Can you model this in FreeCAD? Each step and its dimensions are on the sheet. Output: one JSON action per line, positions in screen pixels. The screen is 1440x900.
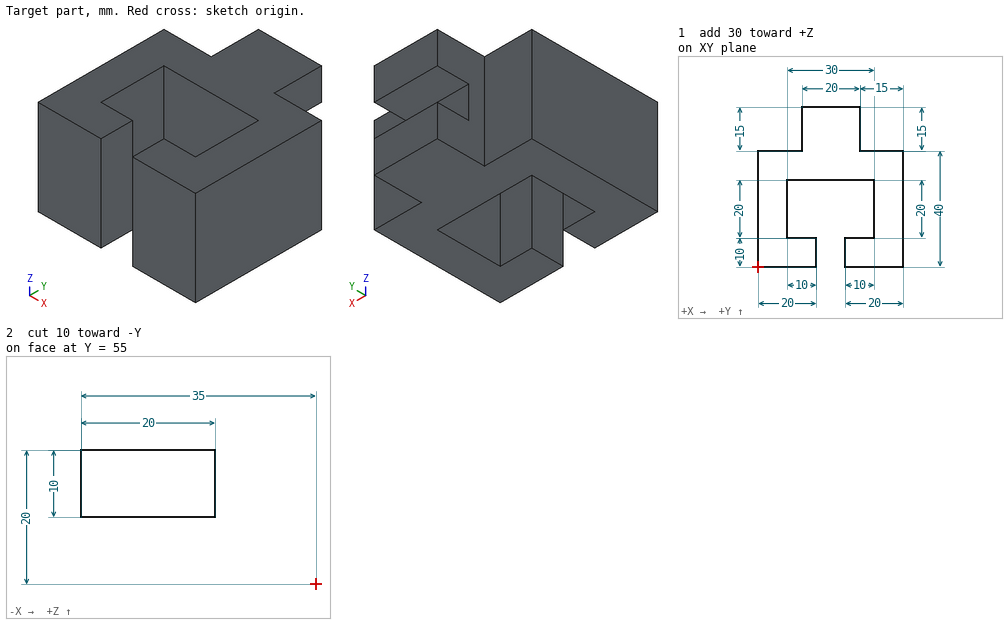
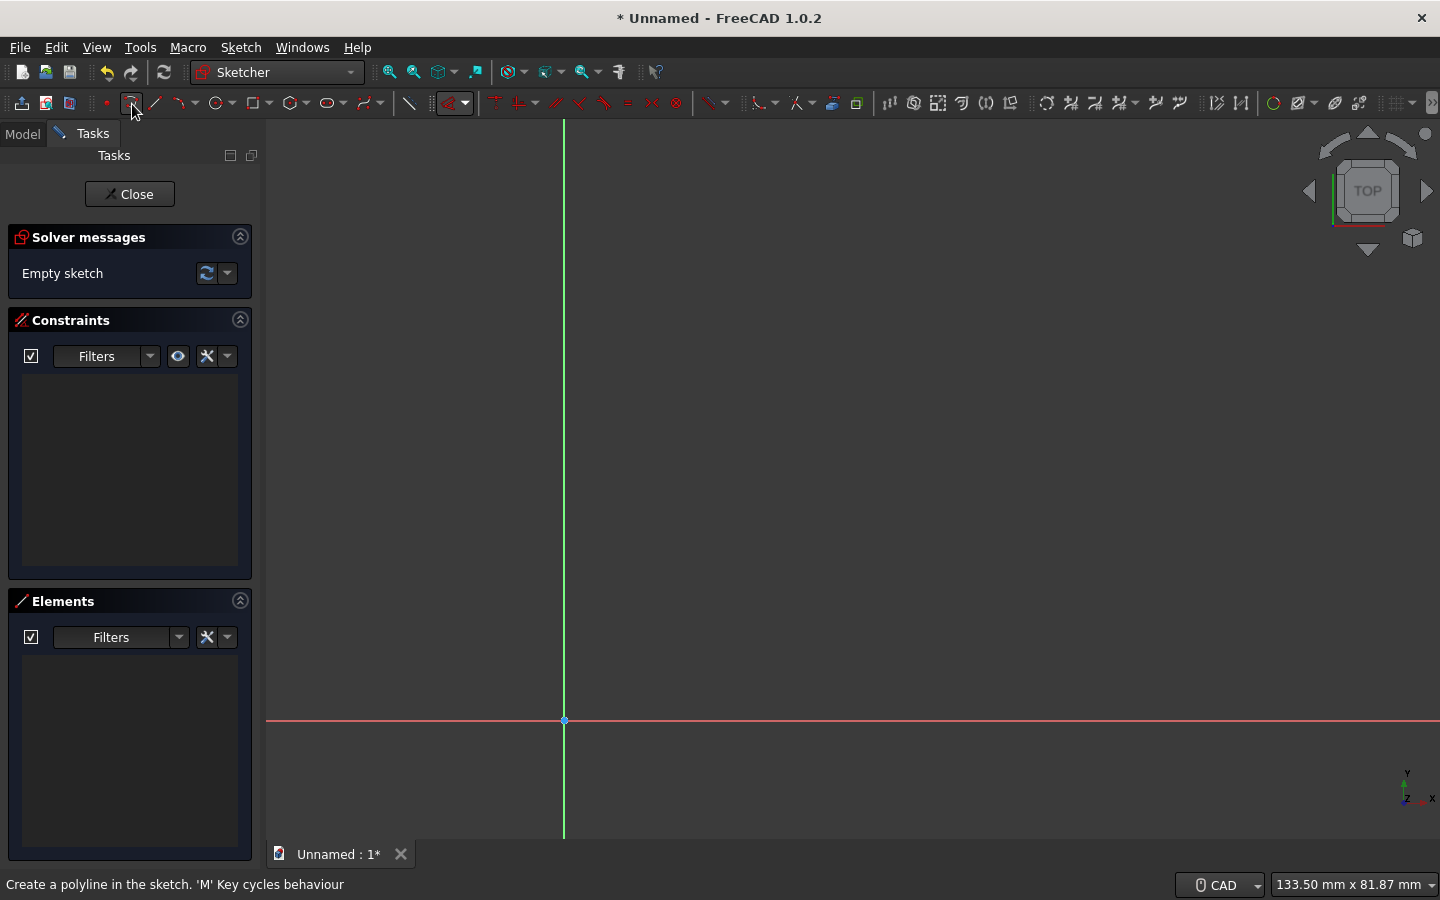
{"action": "left_click", "coordinate": [564, 721]}
{"action": "left_click", "coordinate": [740, 712]}
{"action": "left_click", "coordinate": [740, 633]}
{"action": "left_click", "coordinate": [652, 633]}
{"action": "left_click", "coordinate": [652, 457]}
{"action": "left_click", "coordinate": [916, 457]}
{"action": "left_click", "coordinate": [916, 633]}
{"action": "left_click", "coordinate": [828, 633]}
{"action": "left_click", "coordinate": [828, 721]}
{"action": "left_click", "coordinate": [1004, 712]}
{"action": "left_click", "coordinate": [1004, 369]}
{"action": "left_click", "coordinate": [872, 369]}
{"action": "left_click", "coordinate": [872, 237]}
{"action": "left_click", "coordinate": [696, 237]}
{"action": "left_click", "coordinate": [696, 369]}
{"action": "left_click", "coordinate": [573, 369]}
{"action": "left_click", "coordinate": [564, 721]}
{"action": "key", "text": "Escape"}
{"action": "key", "text": "Escape"}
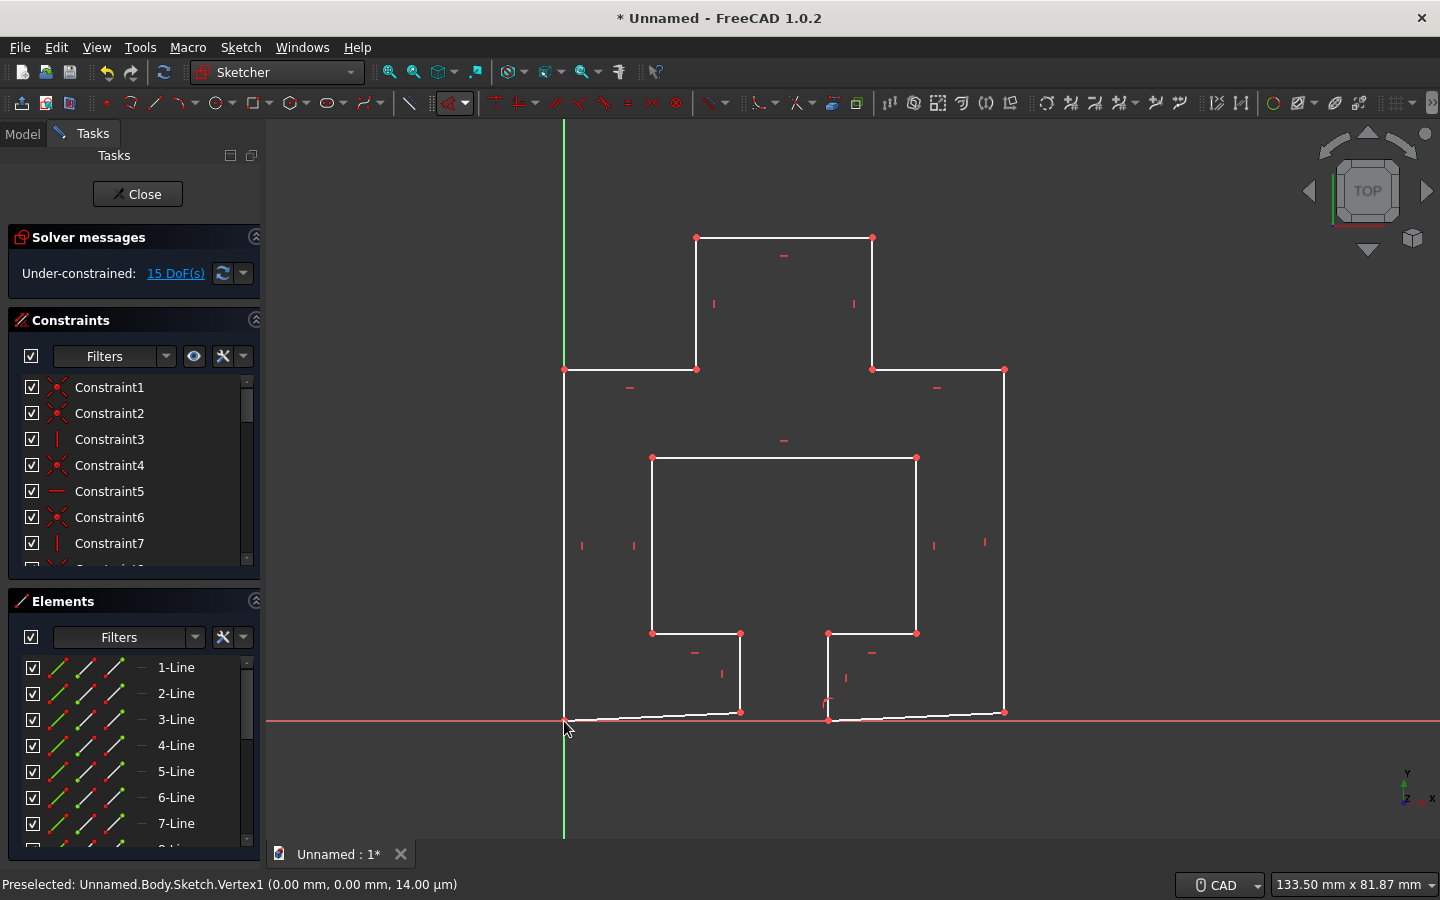
{"action": "left_click", "coordinate": [617, 719]}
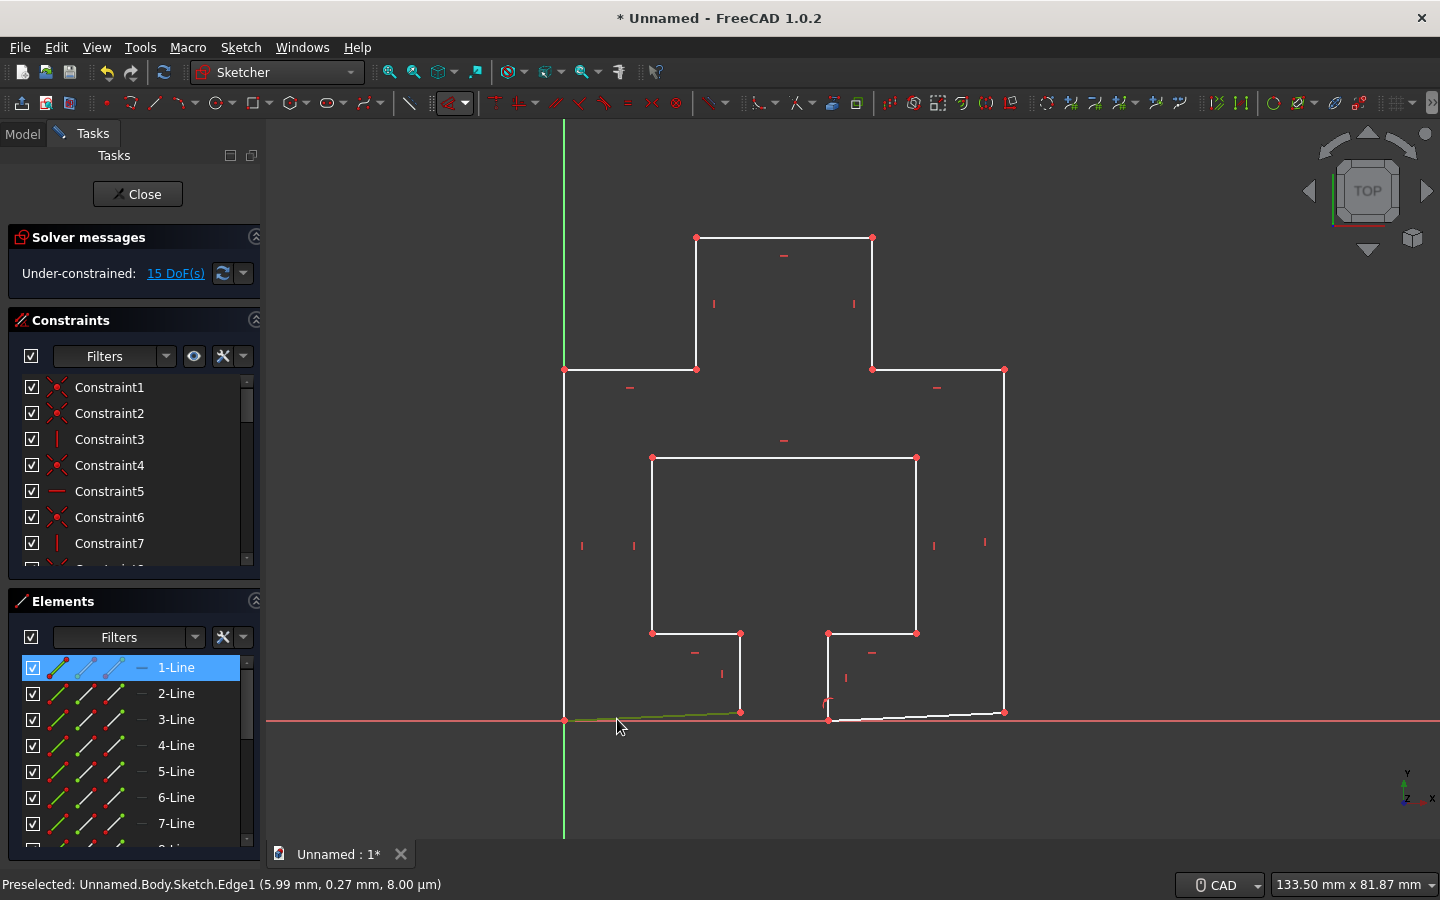
{"action": "key", "text": "h"}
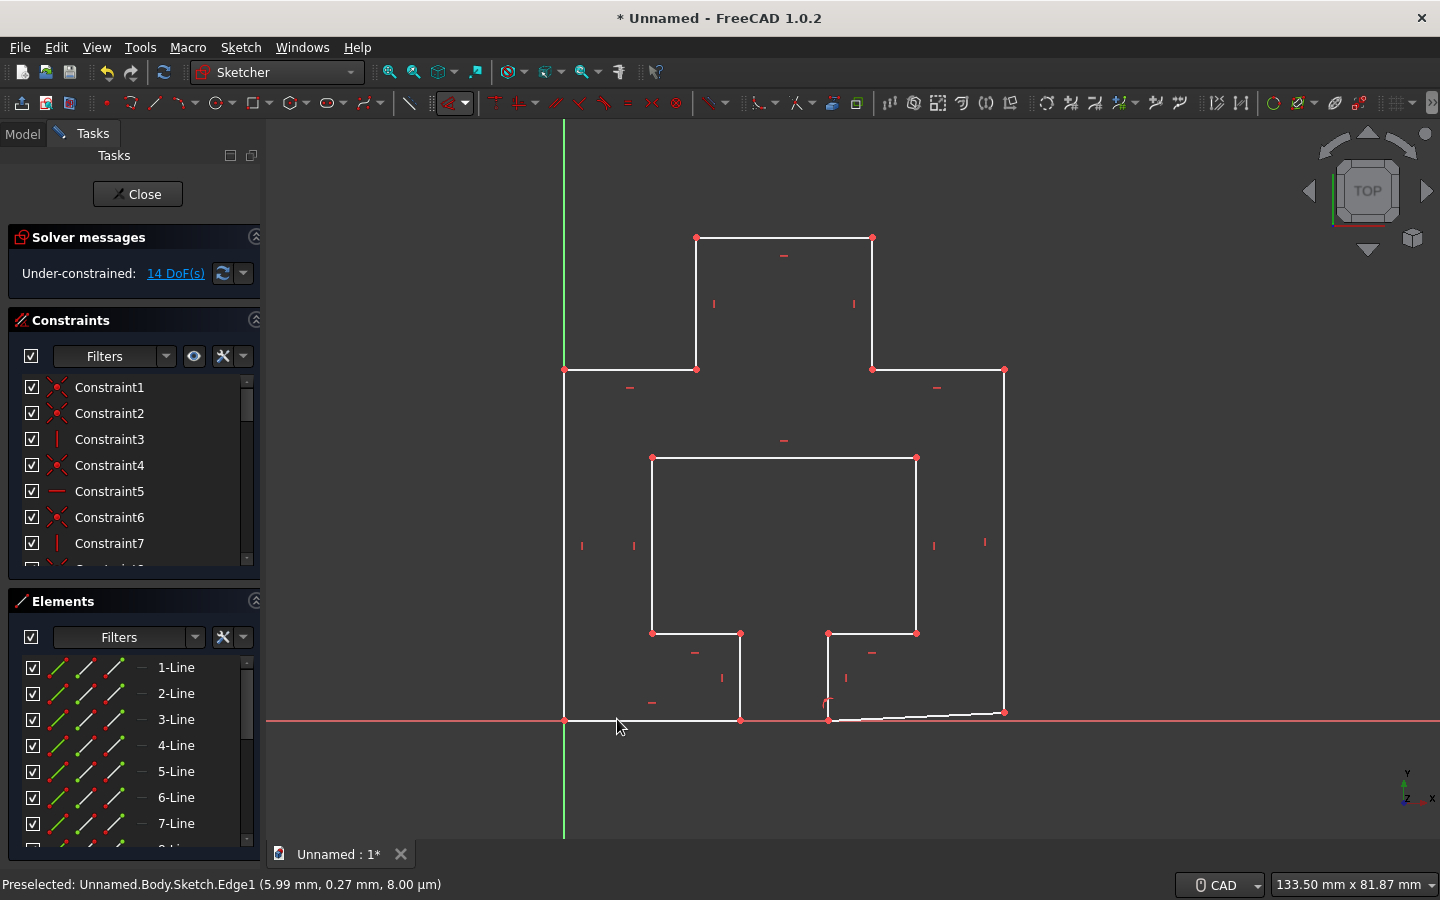
{"action": "left_click", "coordinate": [881, 719]}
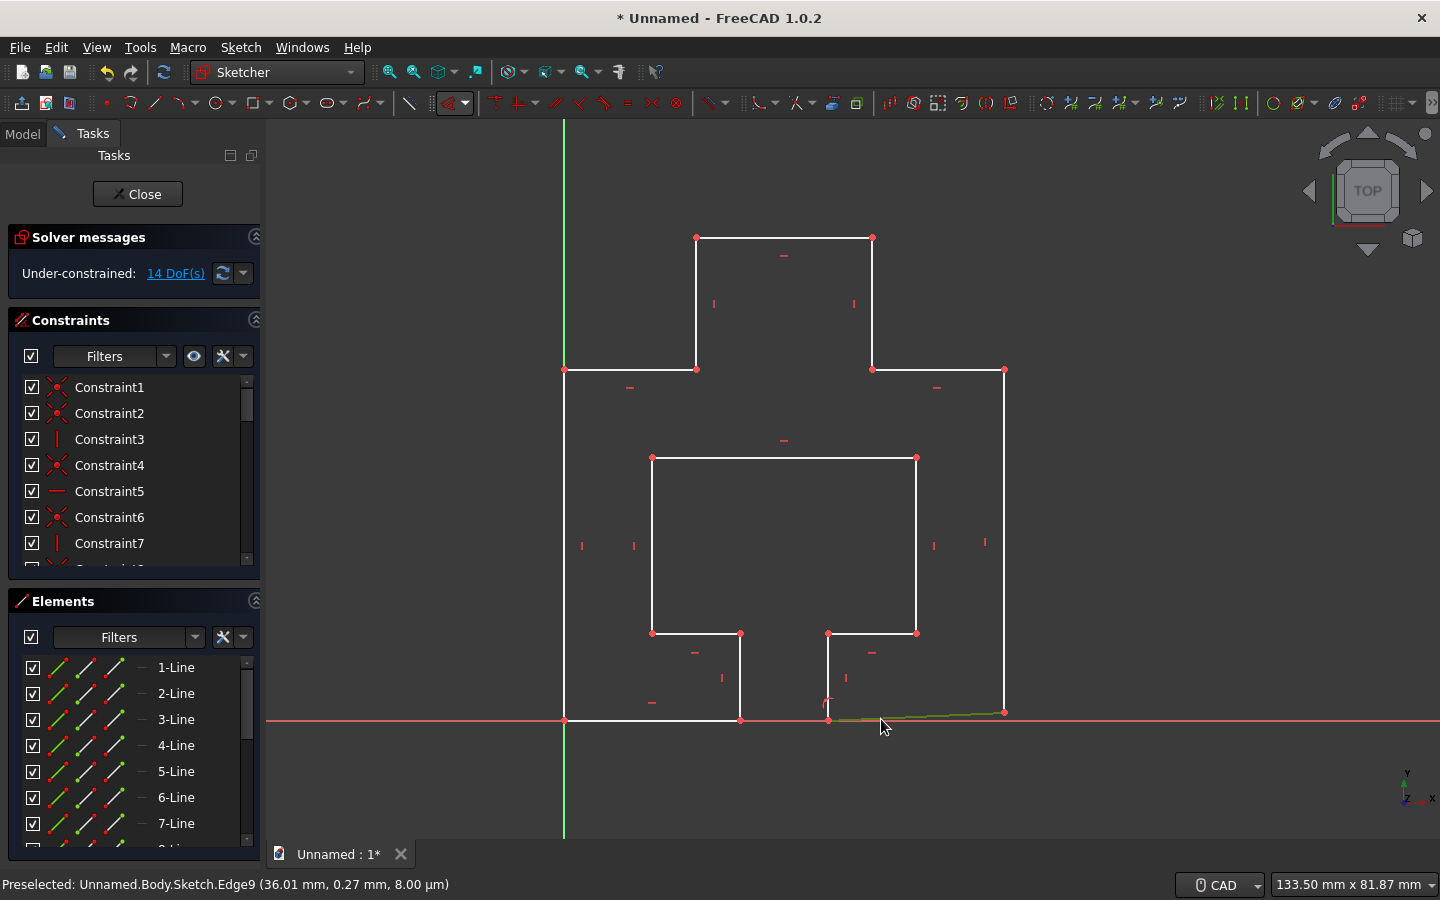
{"action": "key", "text": "h"}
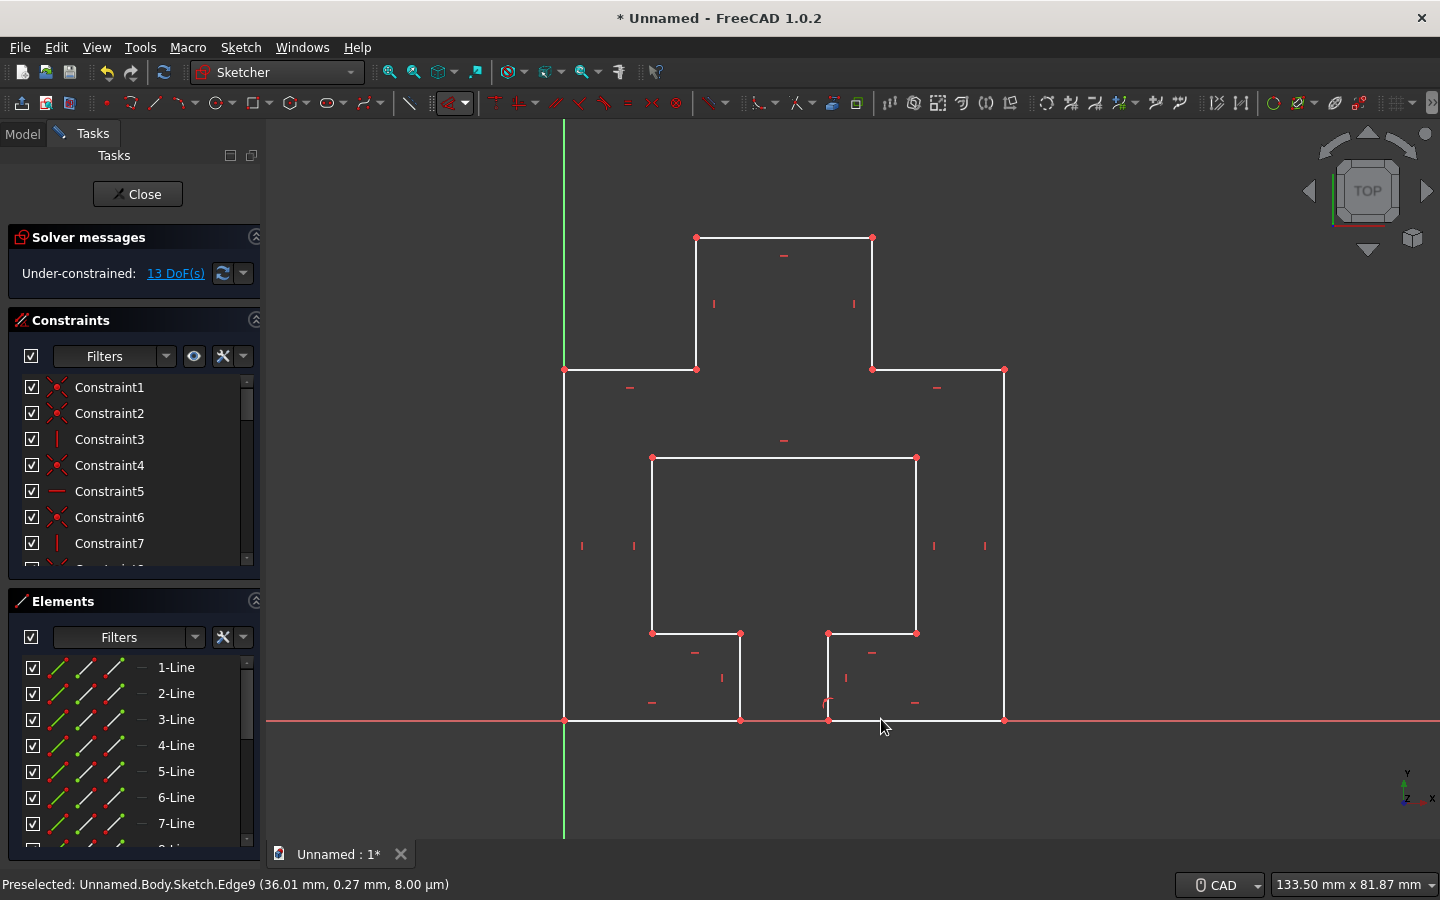
{"action": "key", "text": "d"}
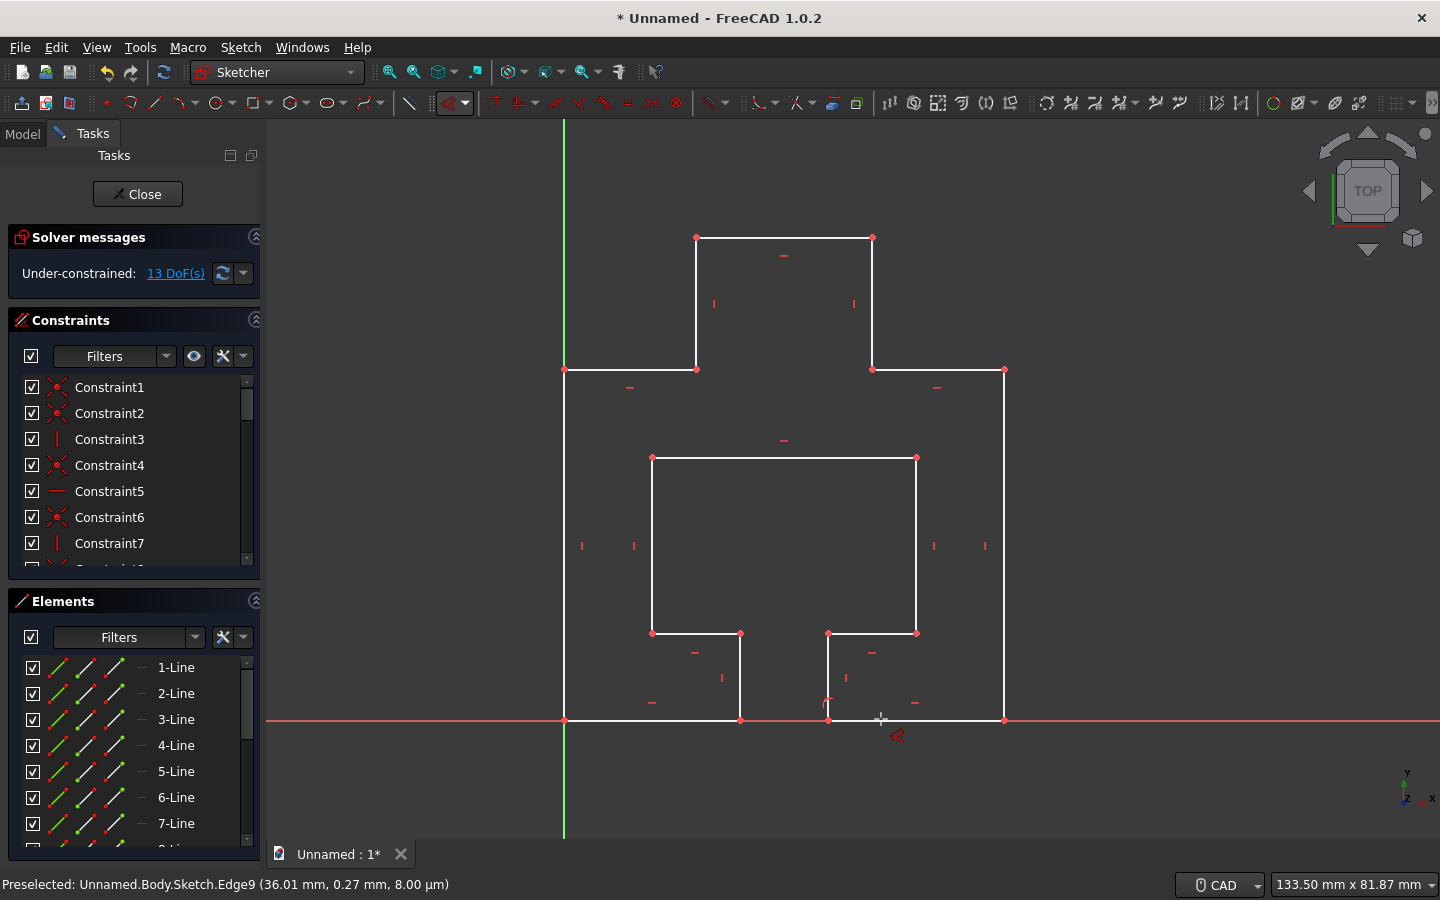
{"action": "left_click", "coordinate": [617, 721]}
{"action": "left_click", "coordinate": [652, 755]}